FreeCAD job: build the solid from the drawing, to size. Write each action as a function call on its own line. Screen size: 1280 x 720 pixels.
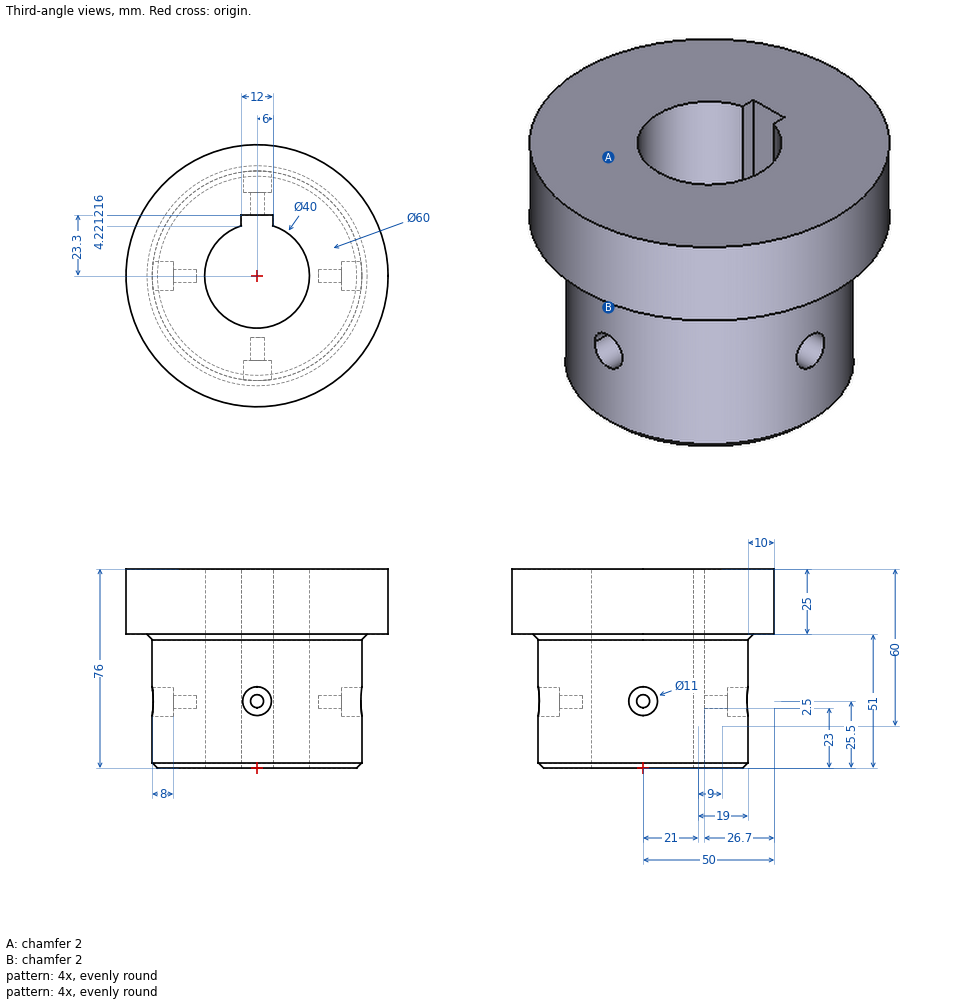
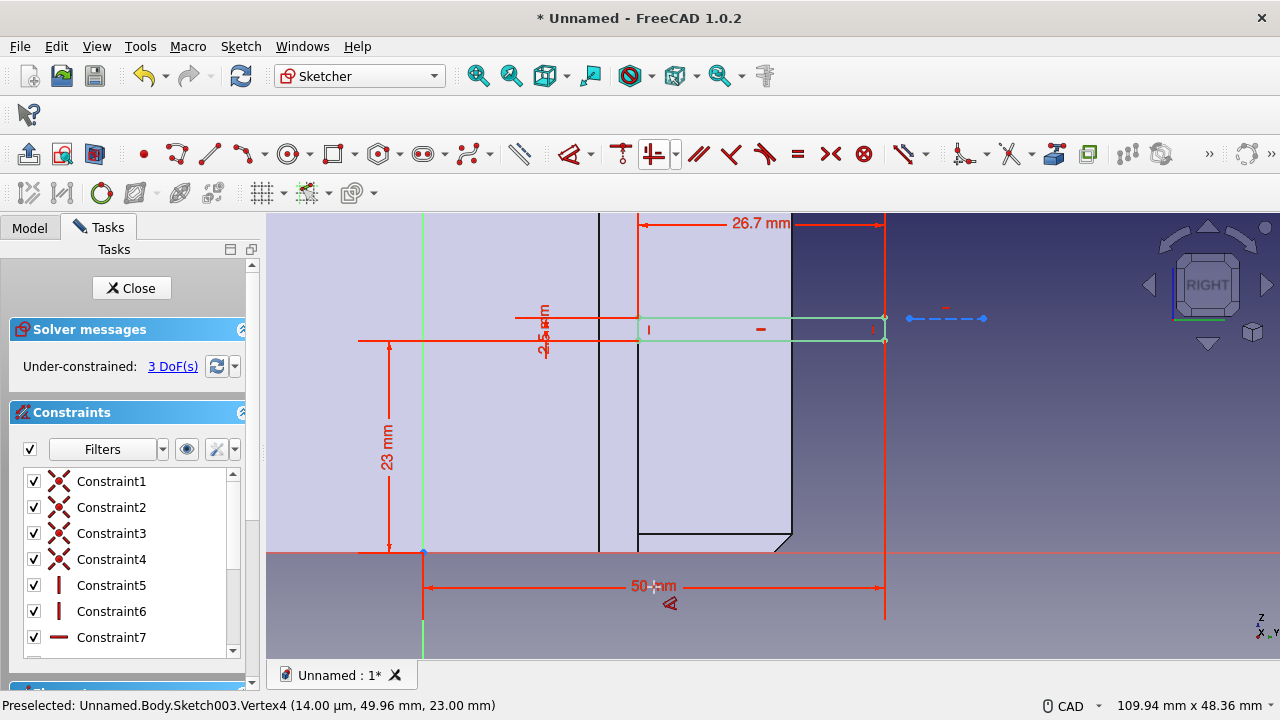
click(909, 319)
click(389, 382)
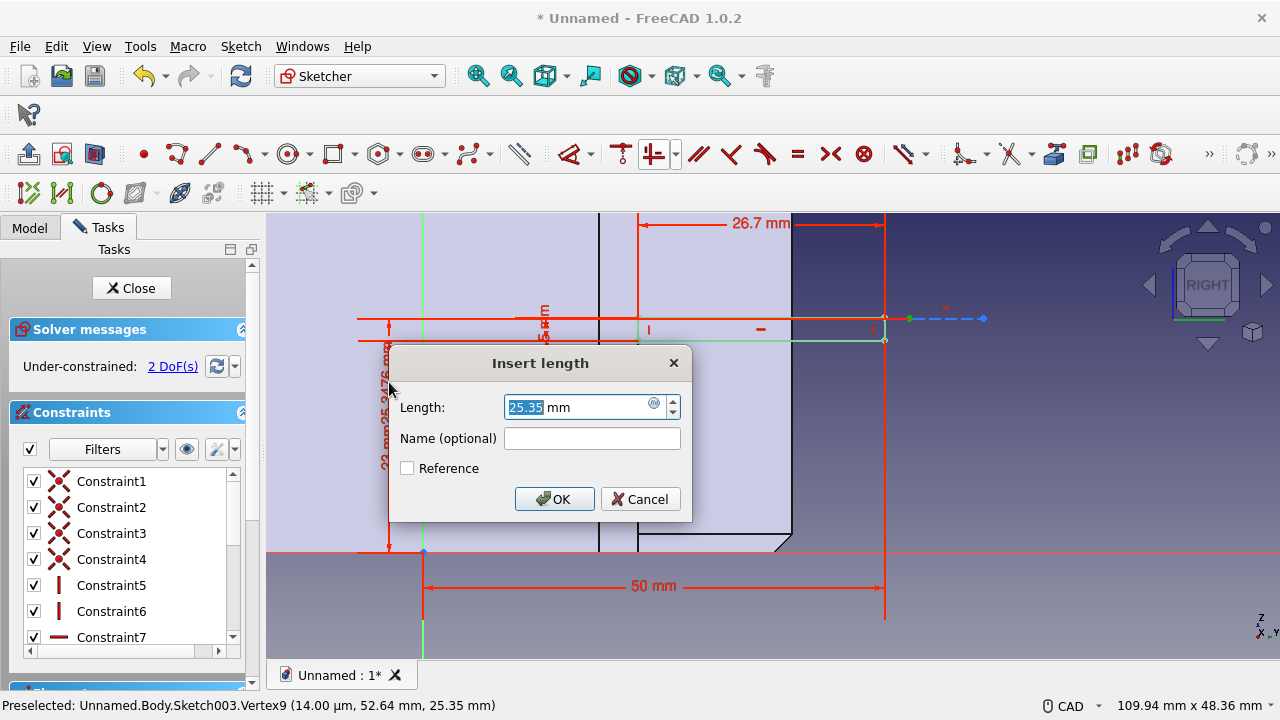
text(25.5)
key(Return)
key(Escape)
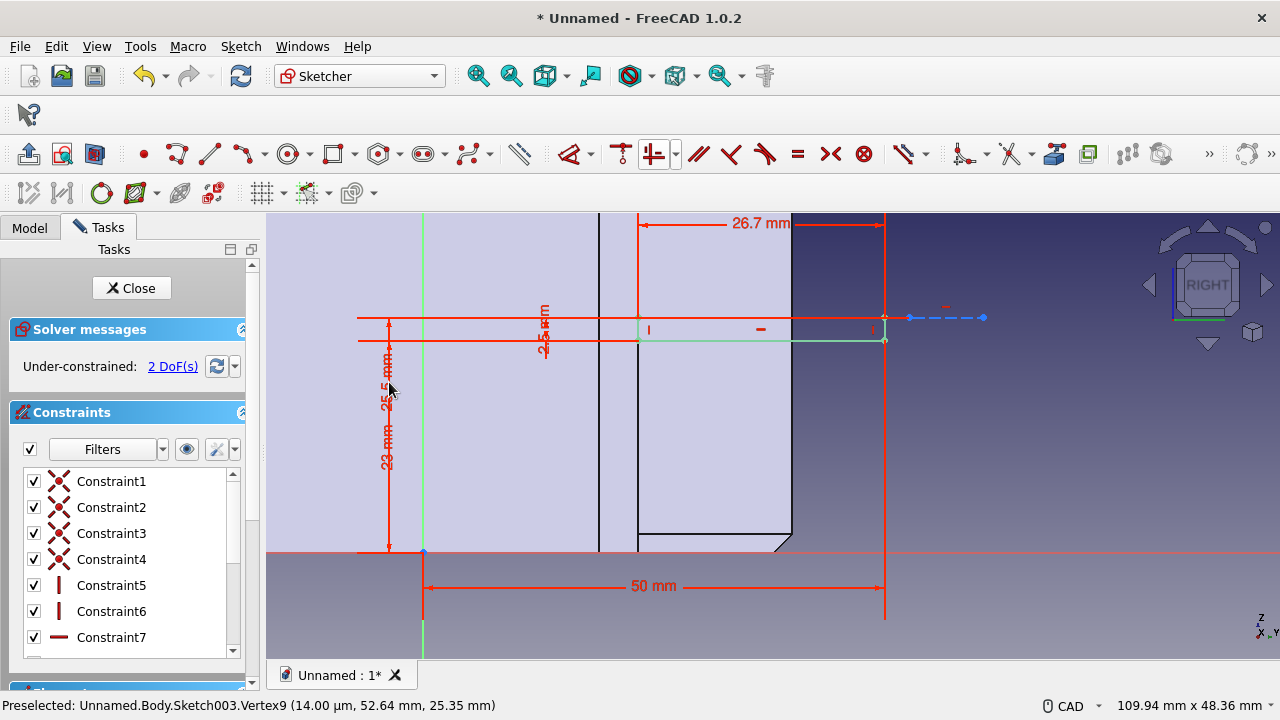
click(132, 288)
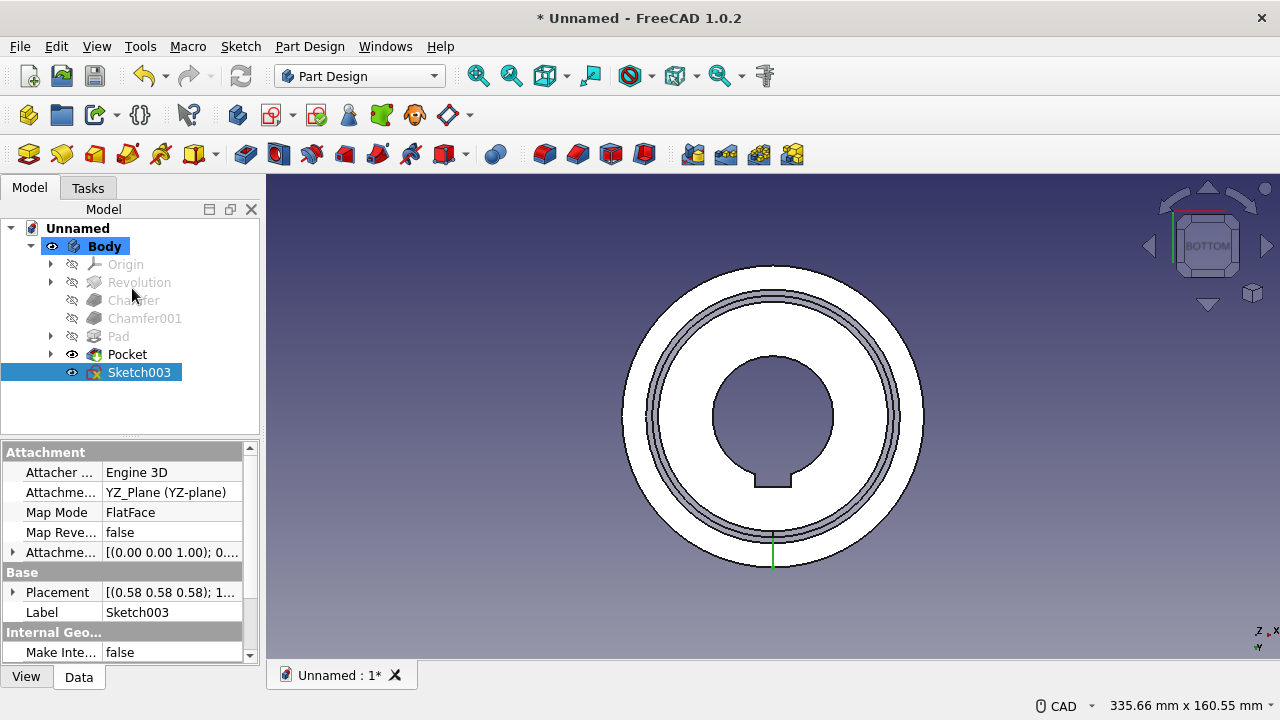
click(312, 154)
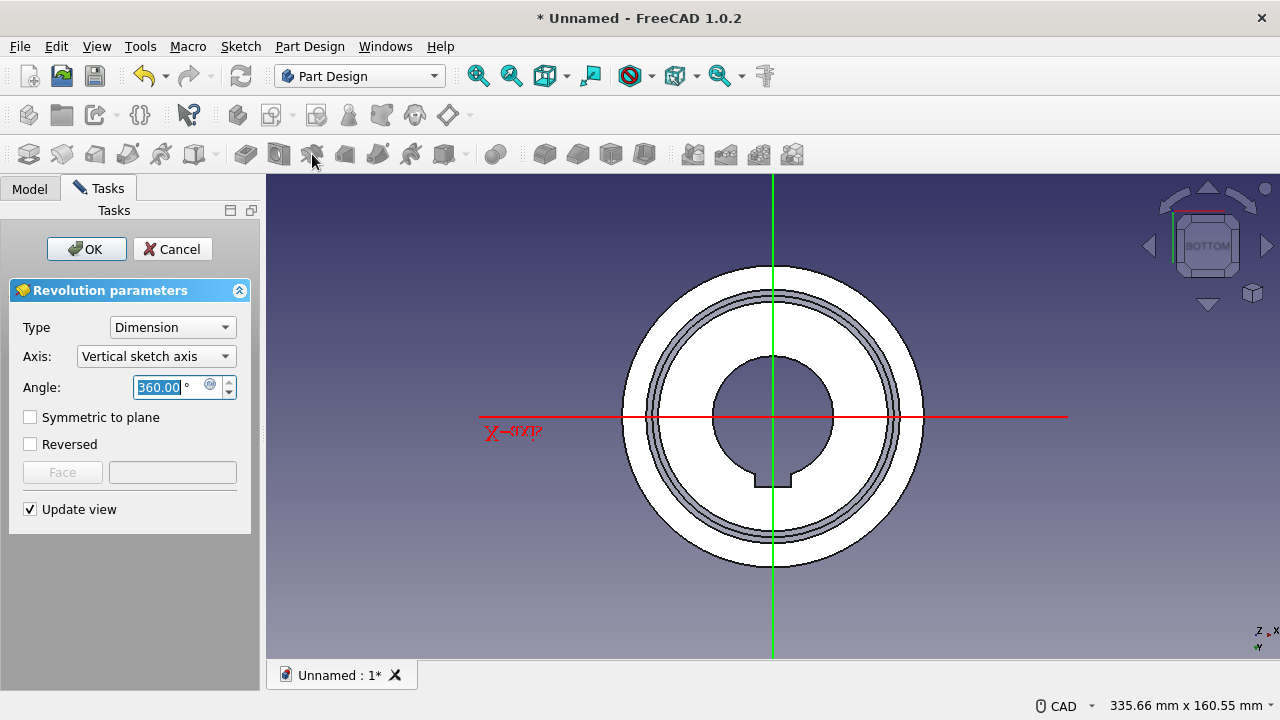
click(157, 356)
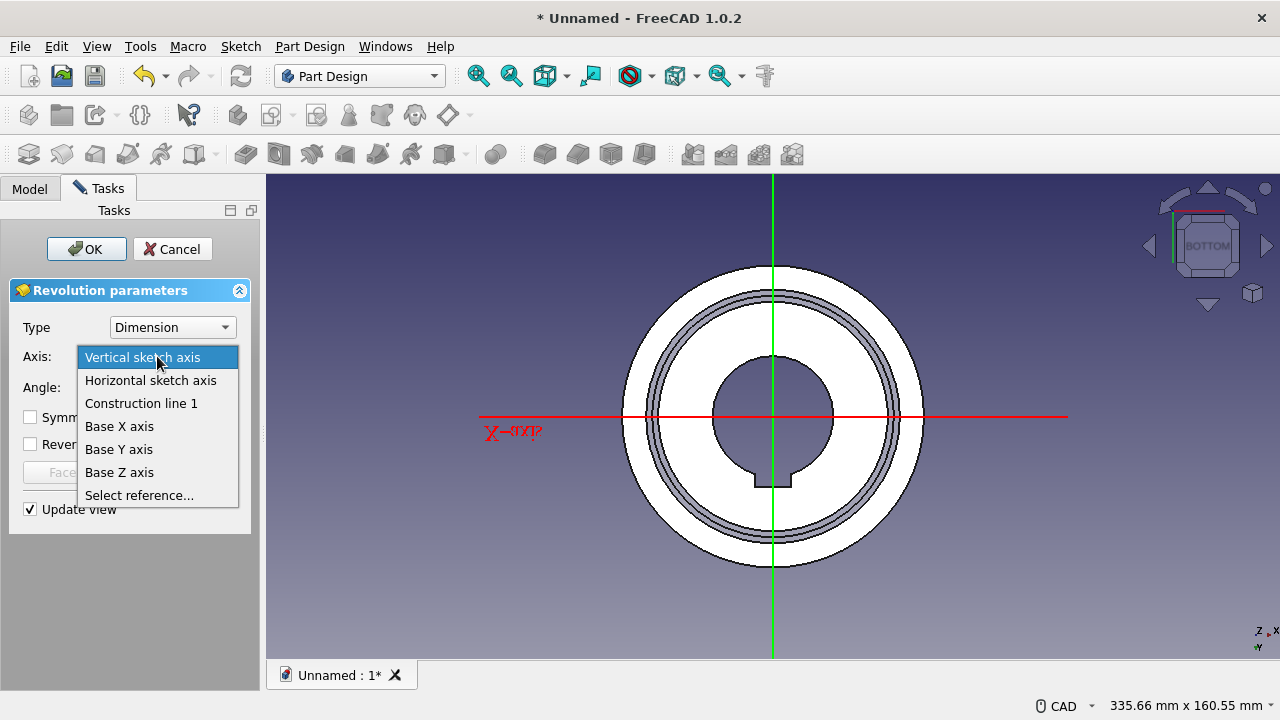
click(156, 404)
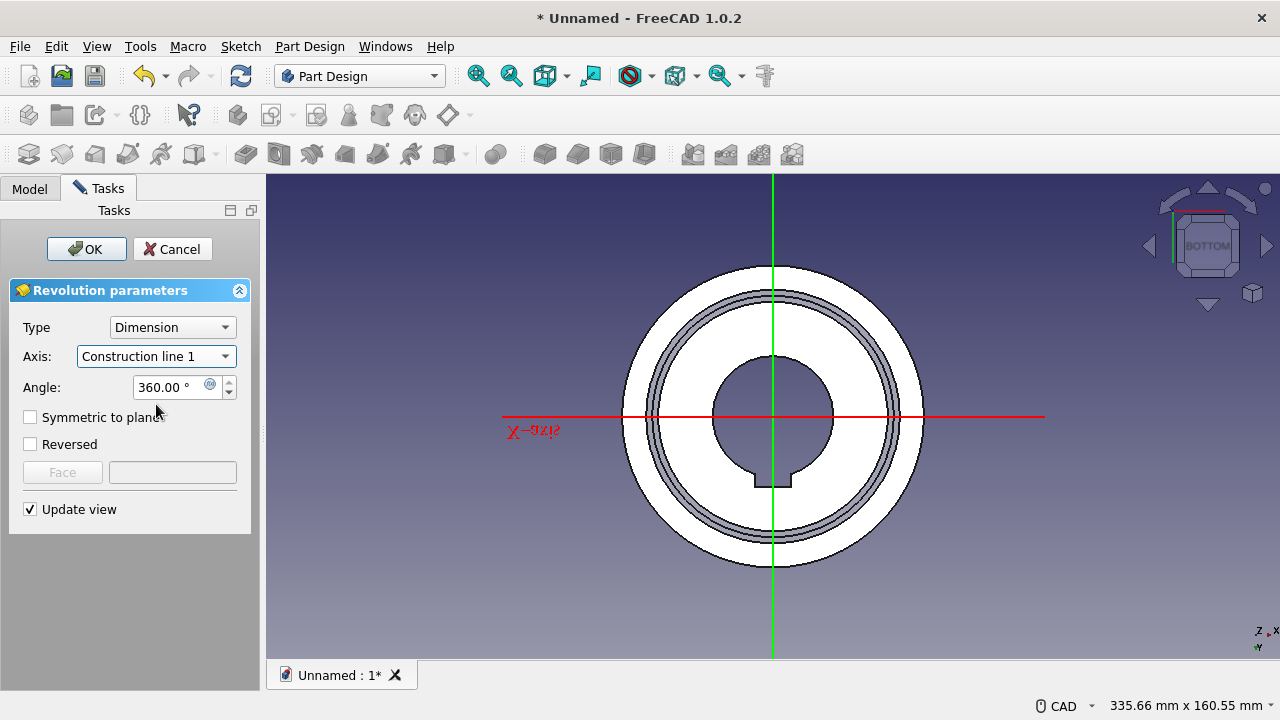
click(87, 249)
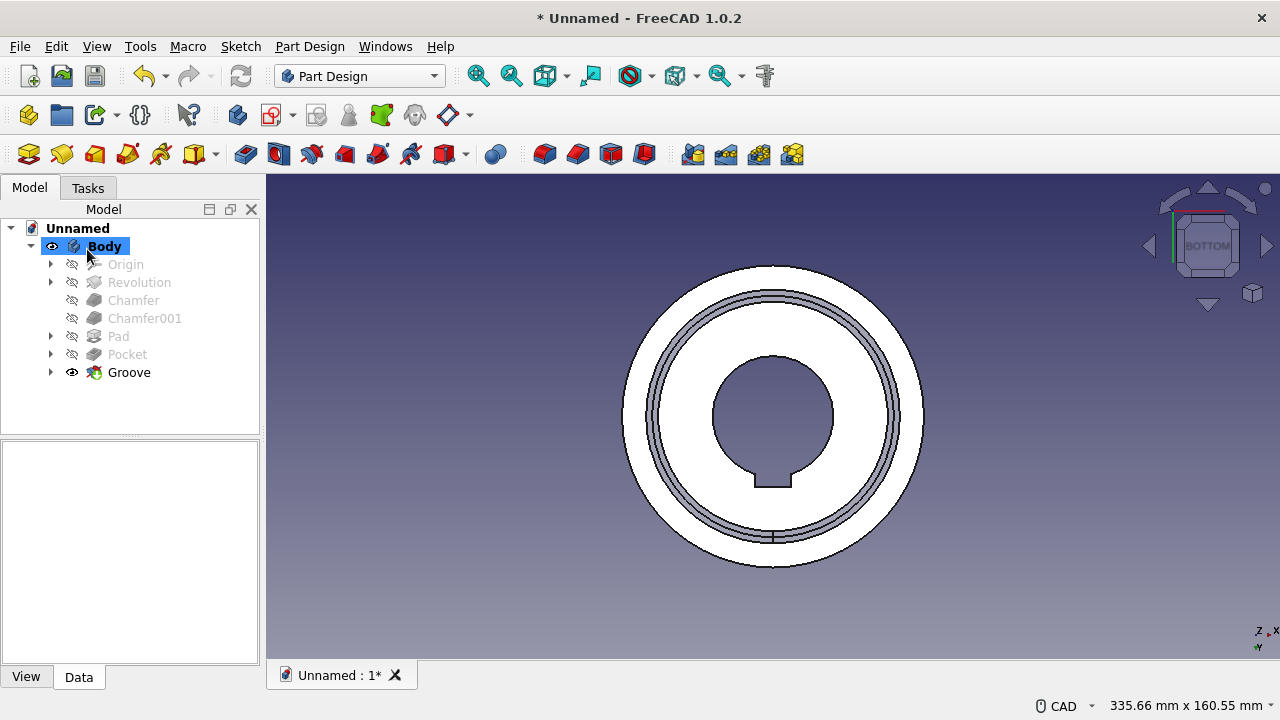
click(117, 372)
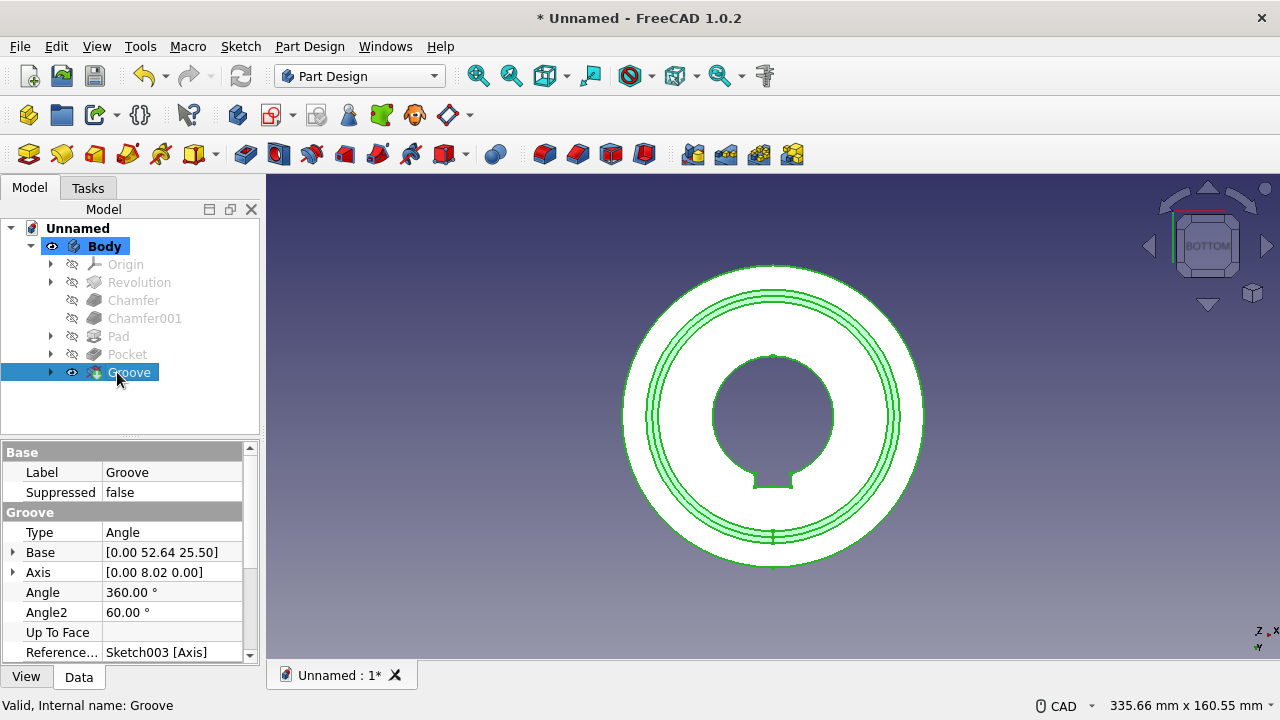
click(759, 154)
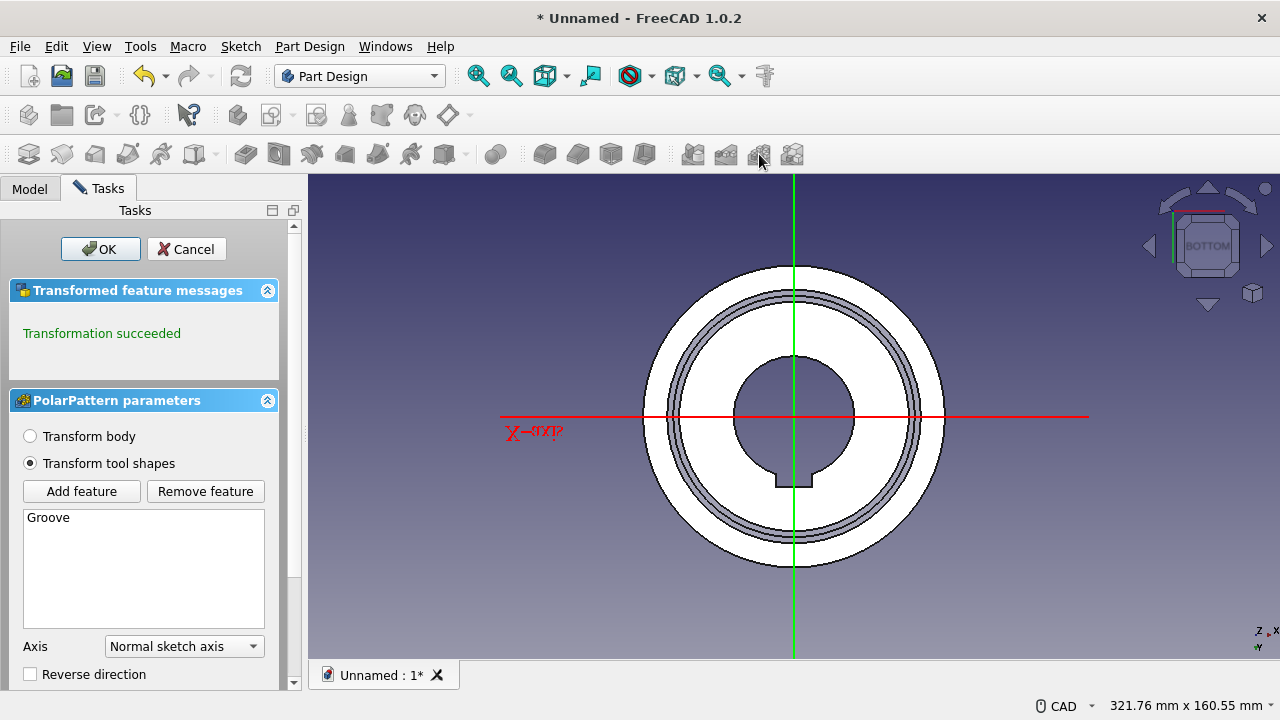
click(185, 646)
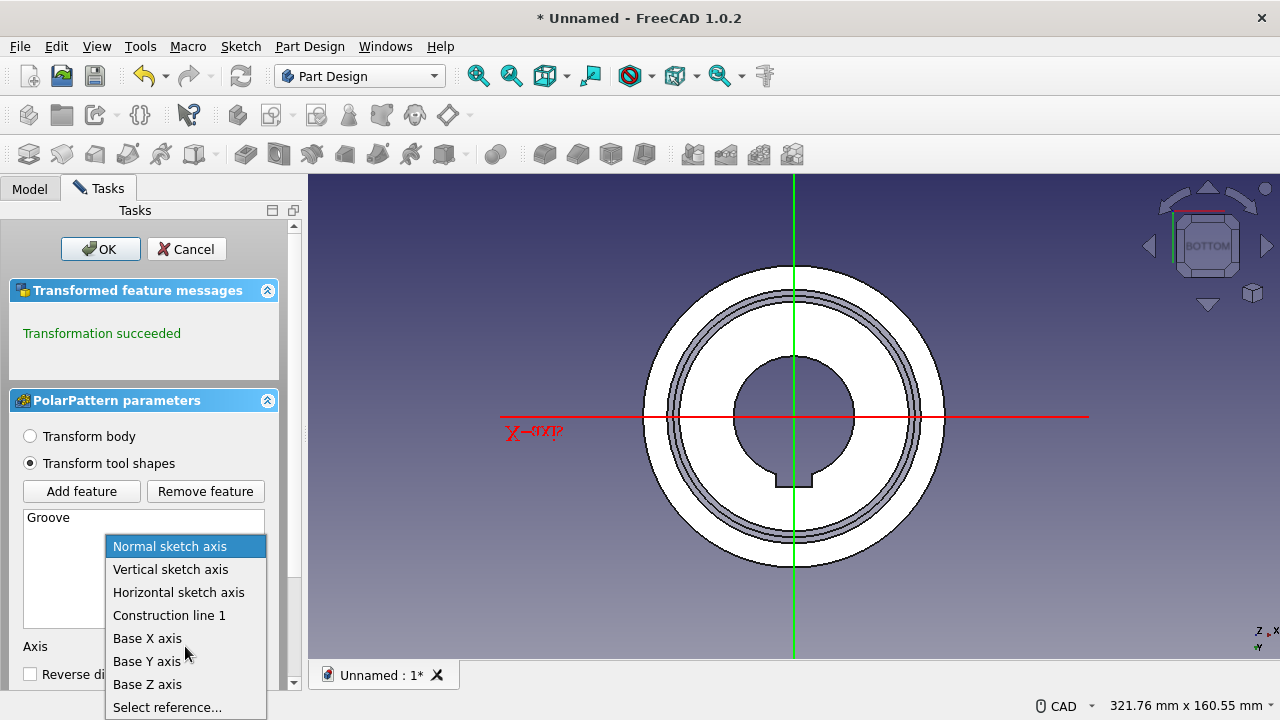
click(184, 684)